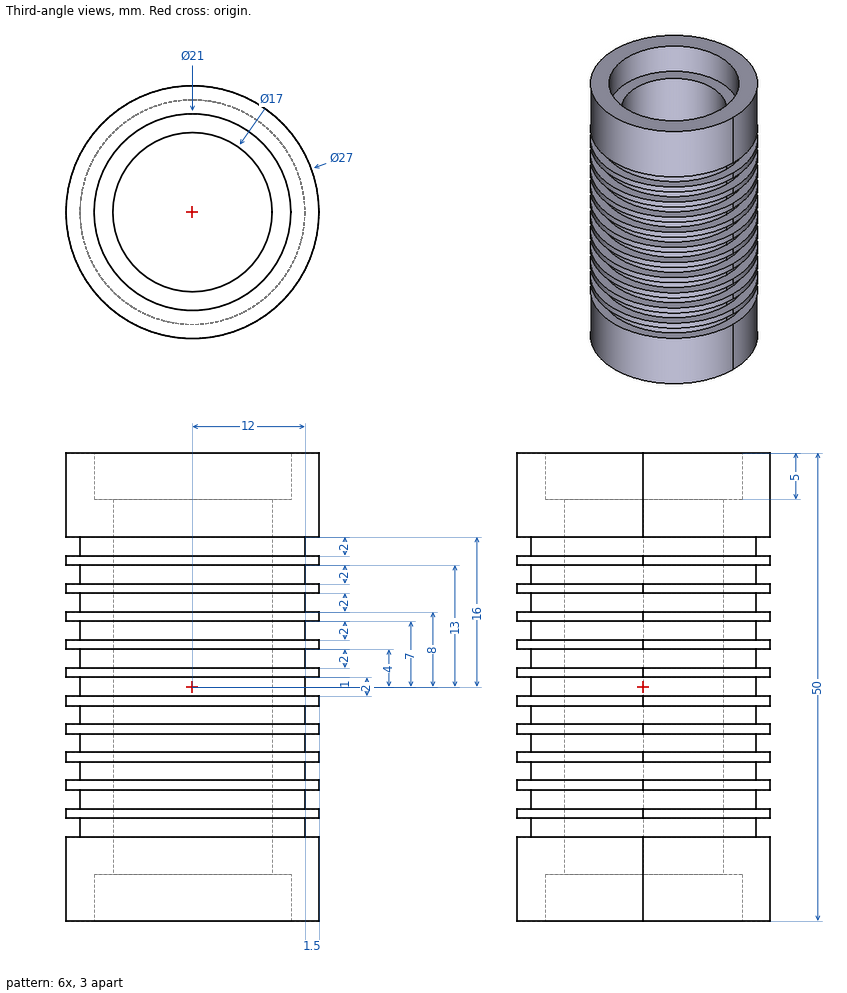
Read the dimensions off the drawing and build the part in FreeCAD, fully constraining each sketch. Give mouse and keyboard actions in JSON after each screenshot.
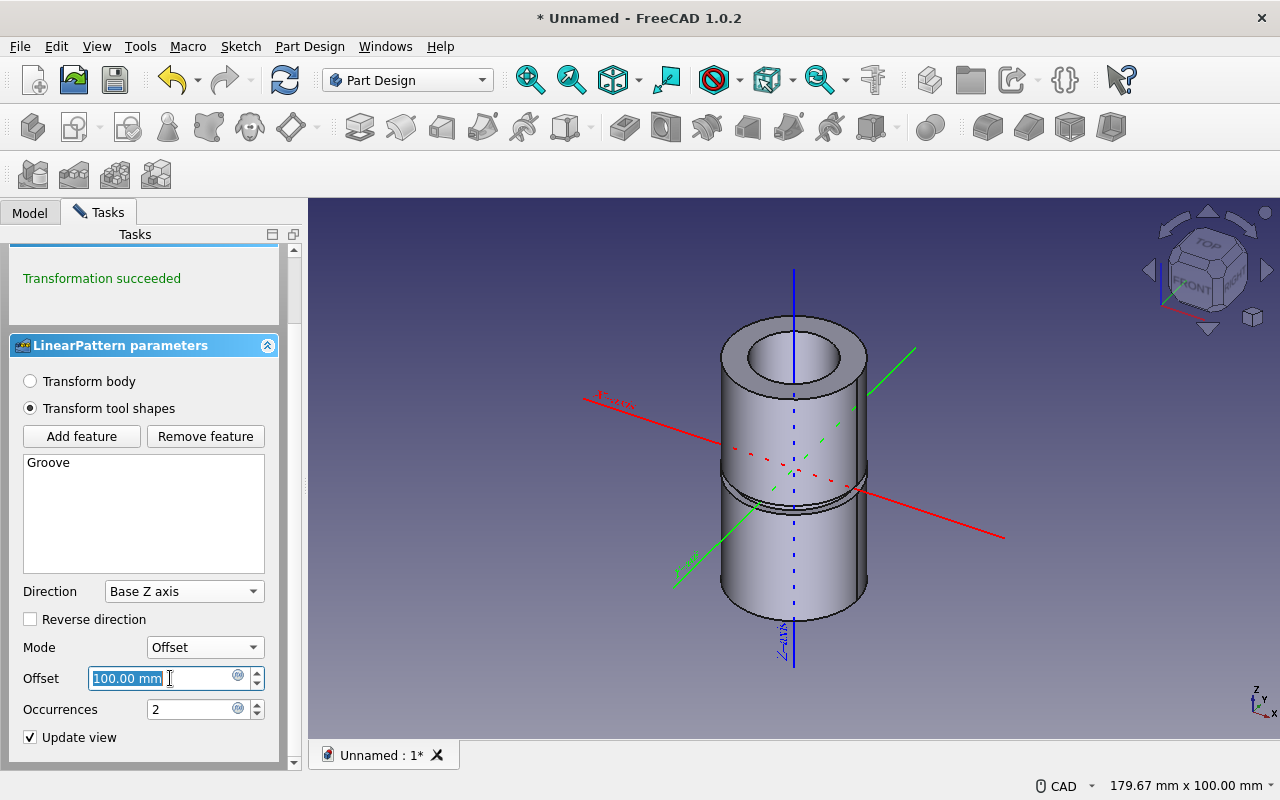
{"action": "type", "text": "3"}
{"action": "key", "text": "Tab"}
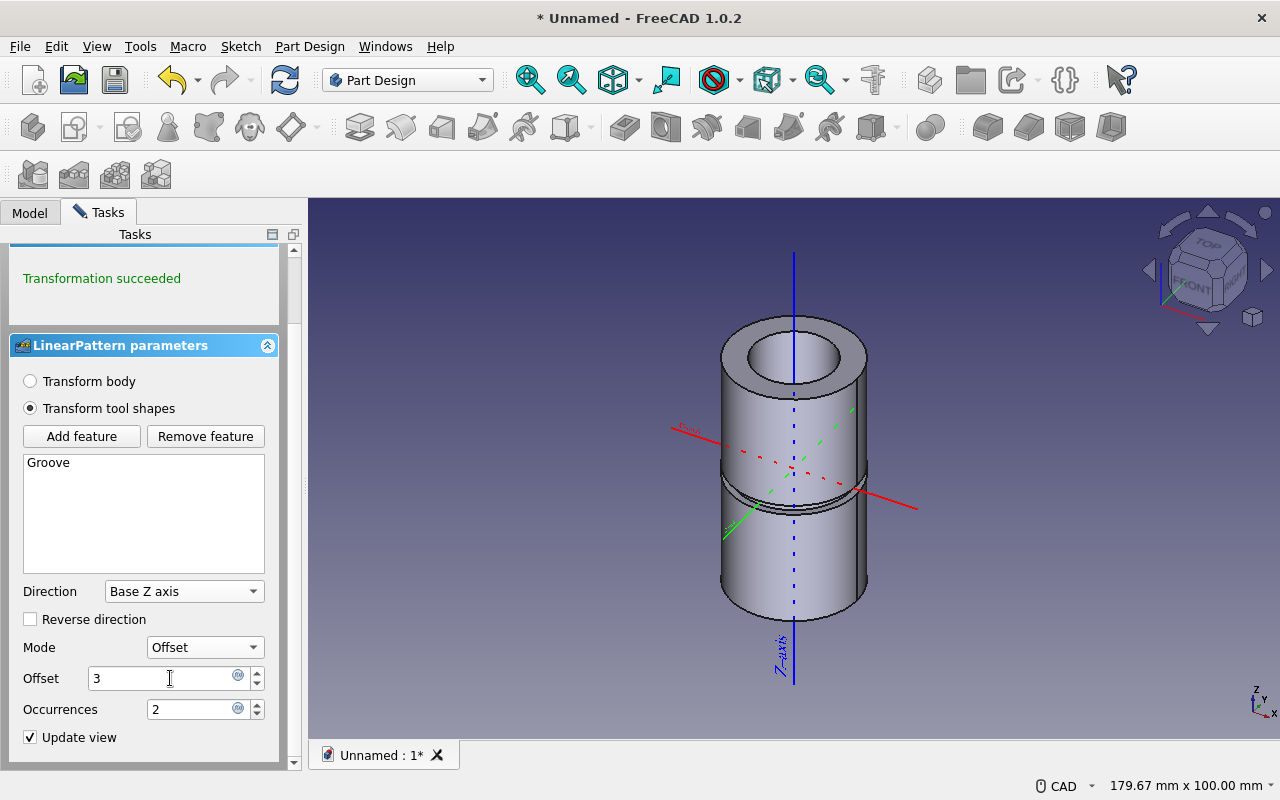
{"action": "triple_click", "coordinate": [199, 710]}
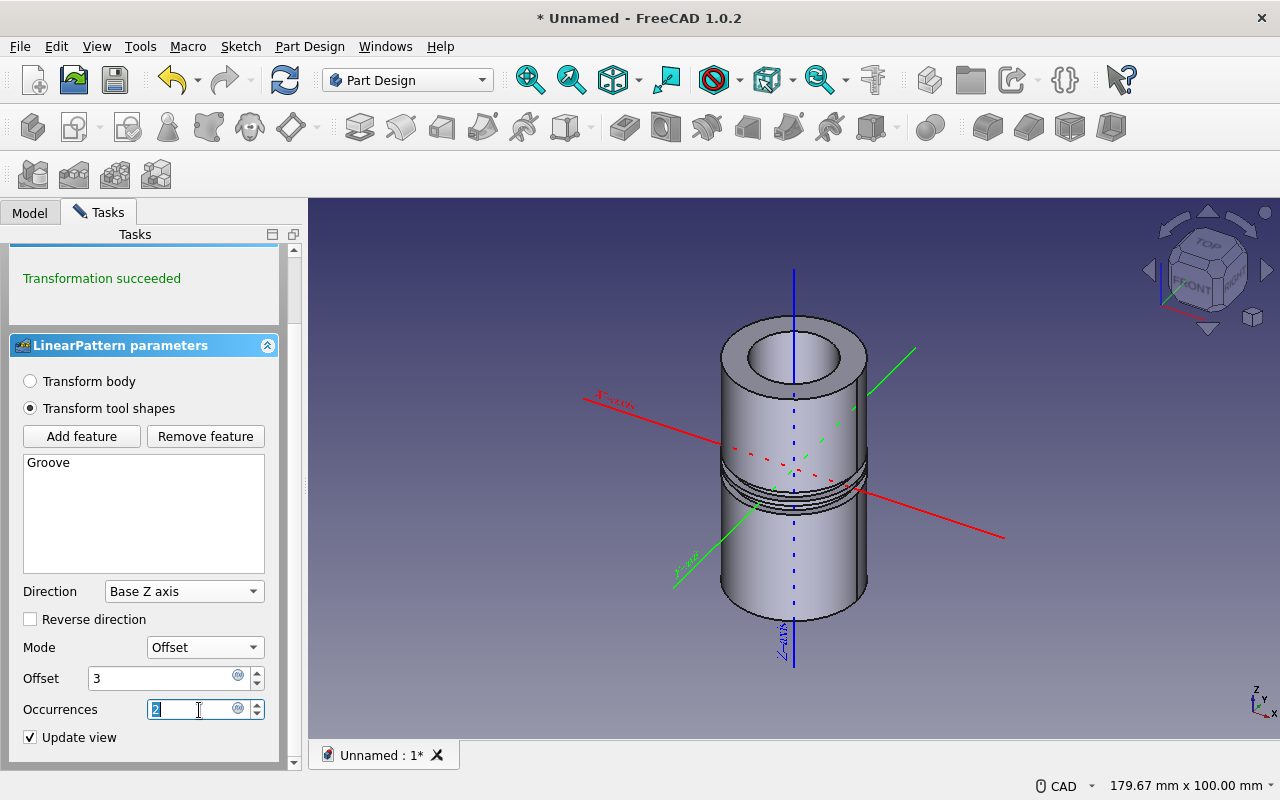
{"action": "type", "text": "6"}
{"action": "key", "text": "Tab"}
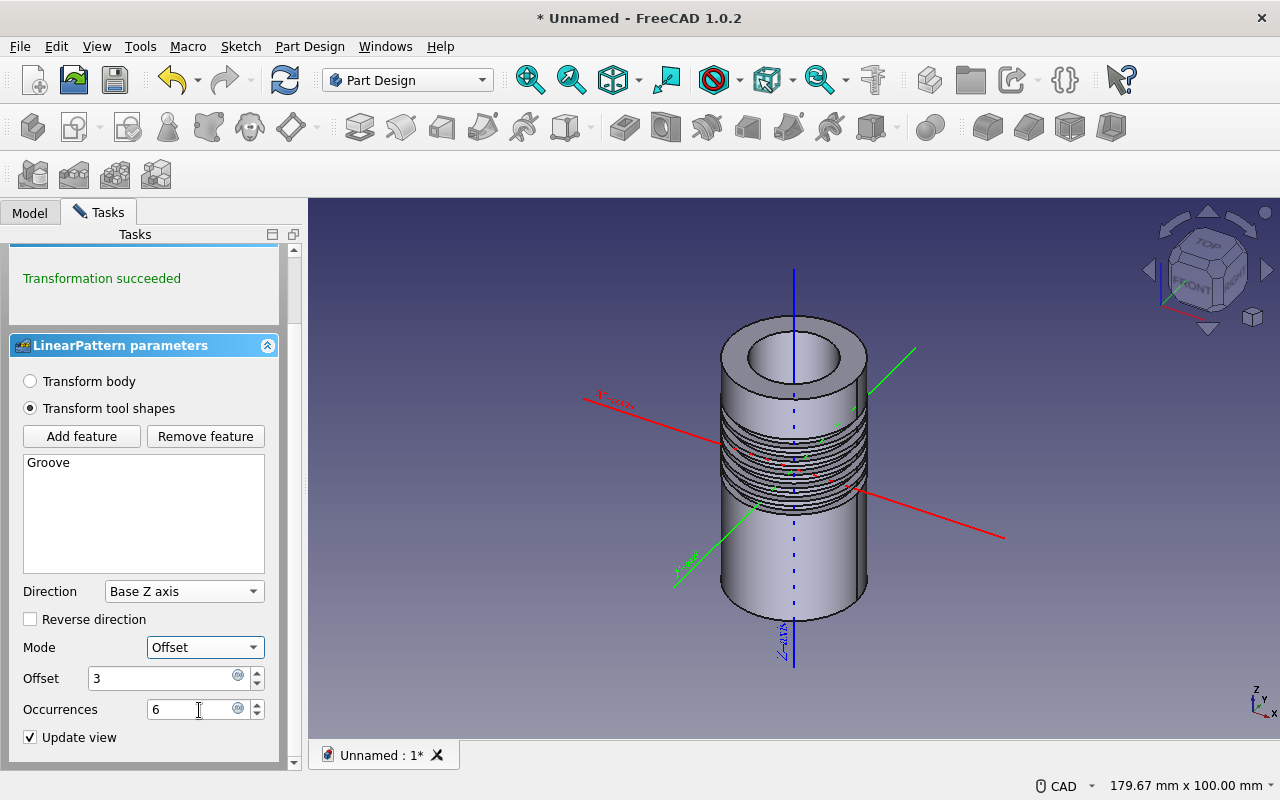
{"action": "left_click", "coordinate": [31, 619]}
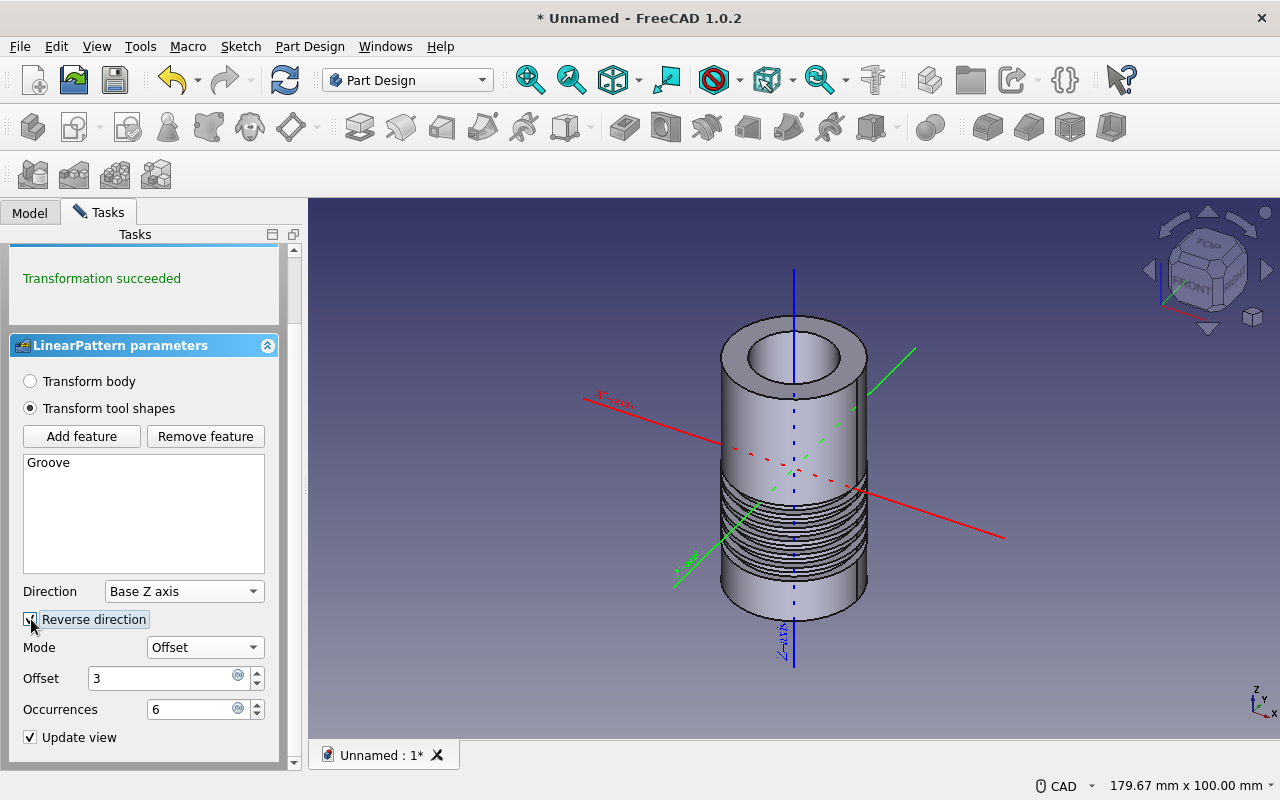
{"action": "scroll", "coordinate": [294, 507], "scroll_direction": "up", "scroll_amount": 3}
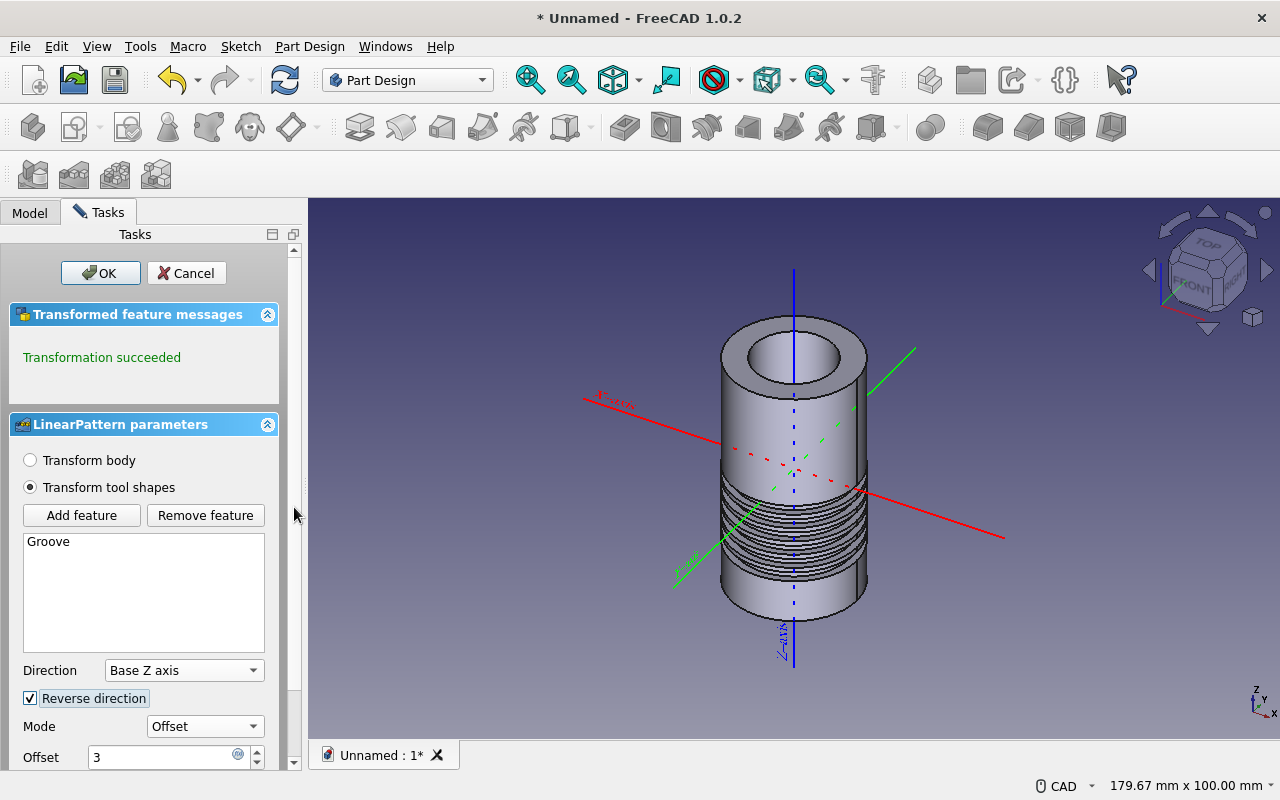
{"action": "left_click", "coordinate": [101, 273]}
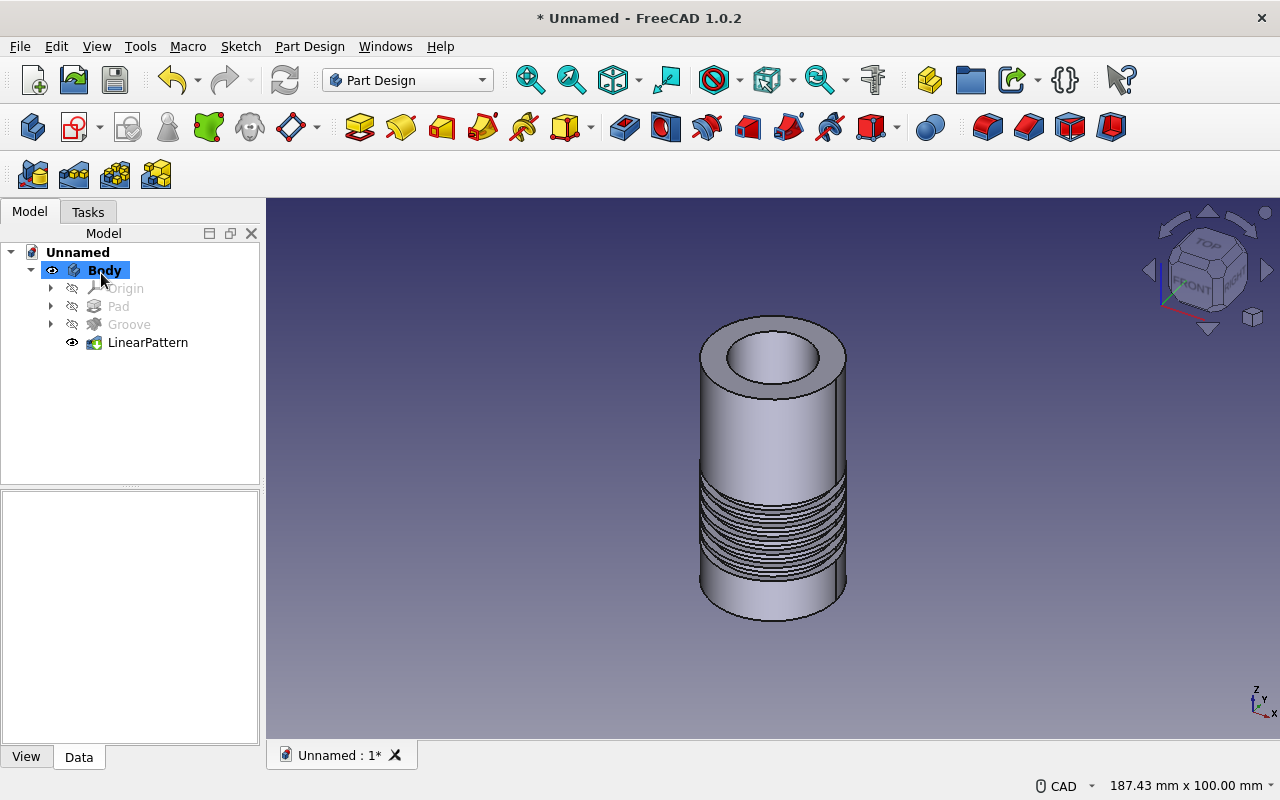
{"action": "left_click", "coordinate": [74, 128]}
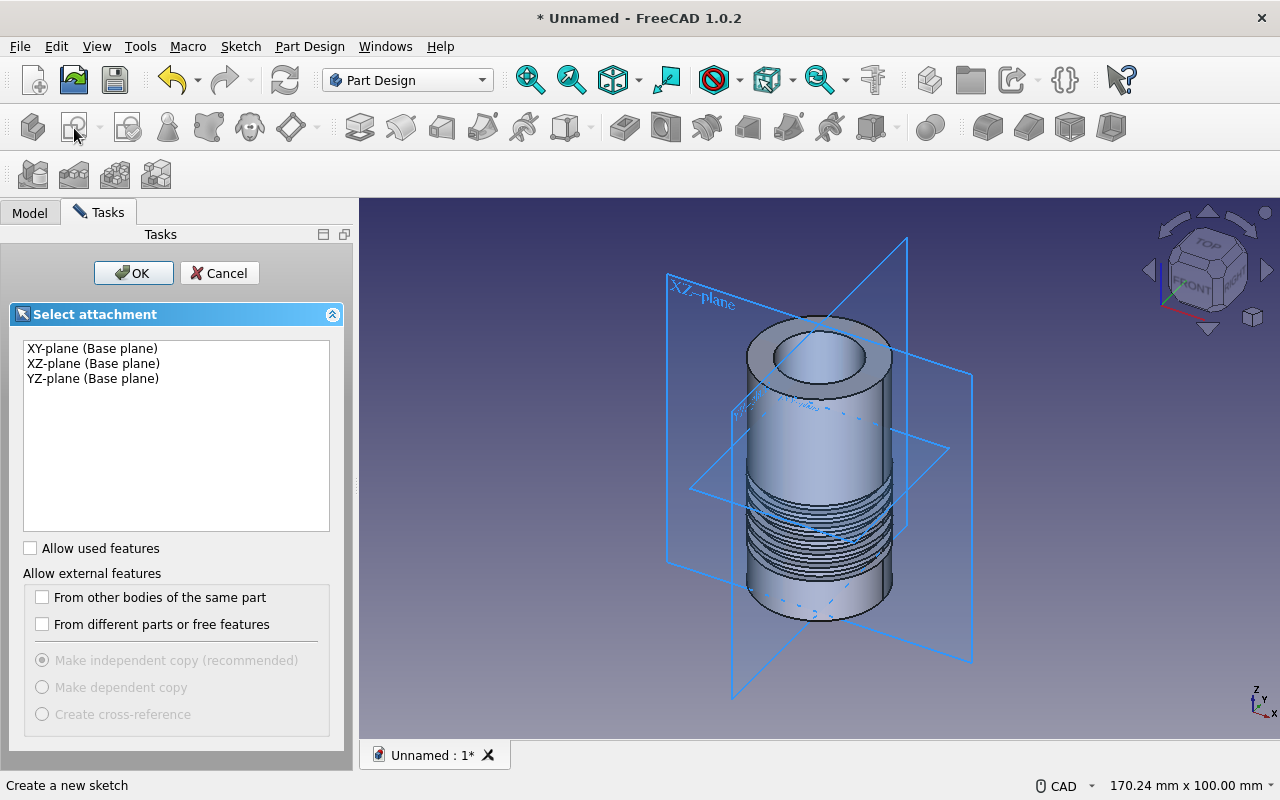
{"action": "left_click", "coordinate": [84, 364]}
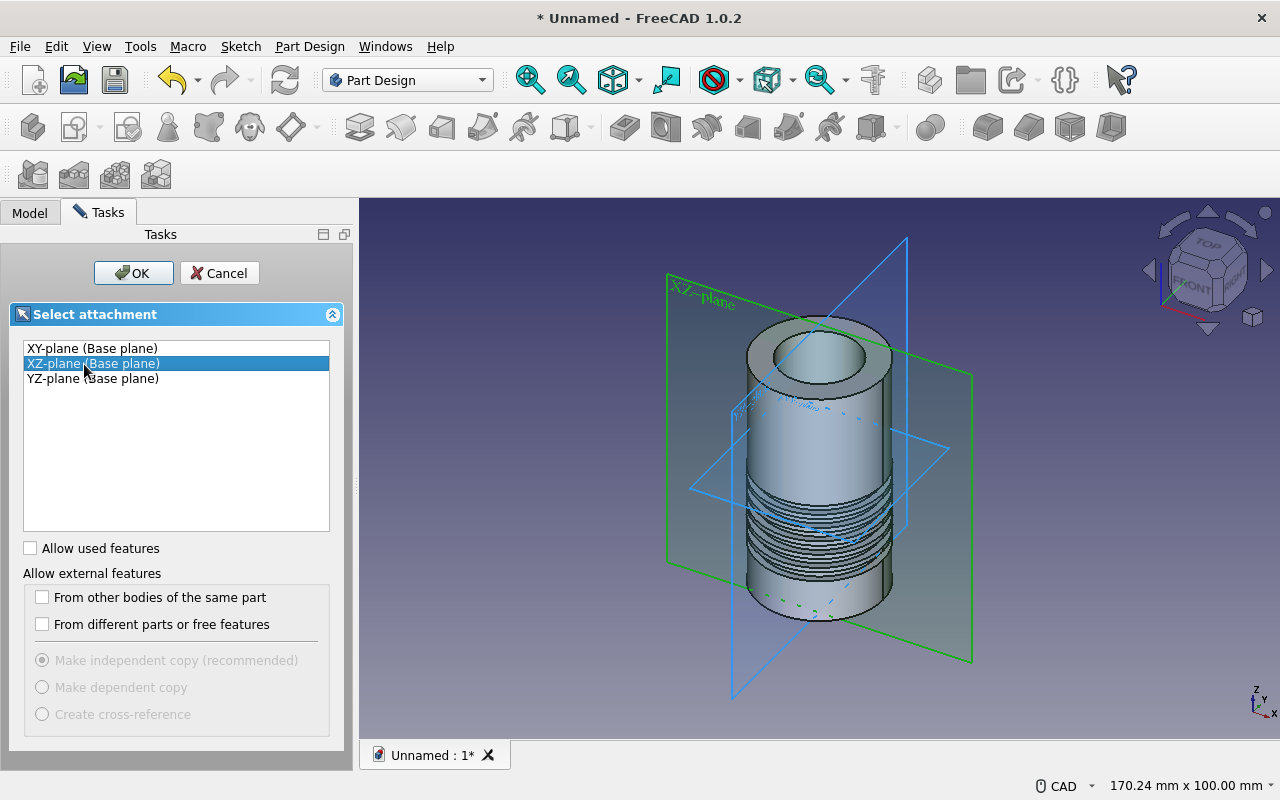
{"action": "left_click", "coordinate": [134, 273]}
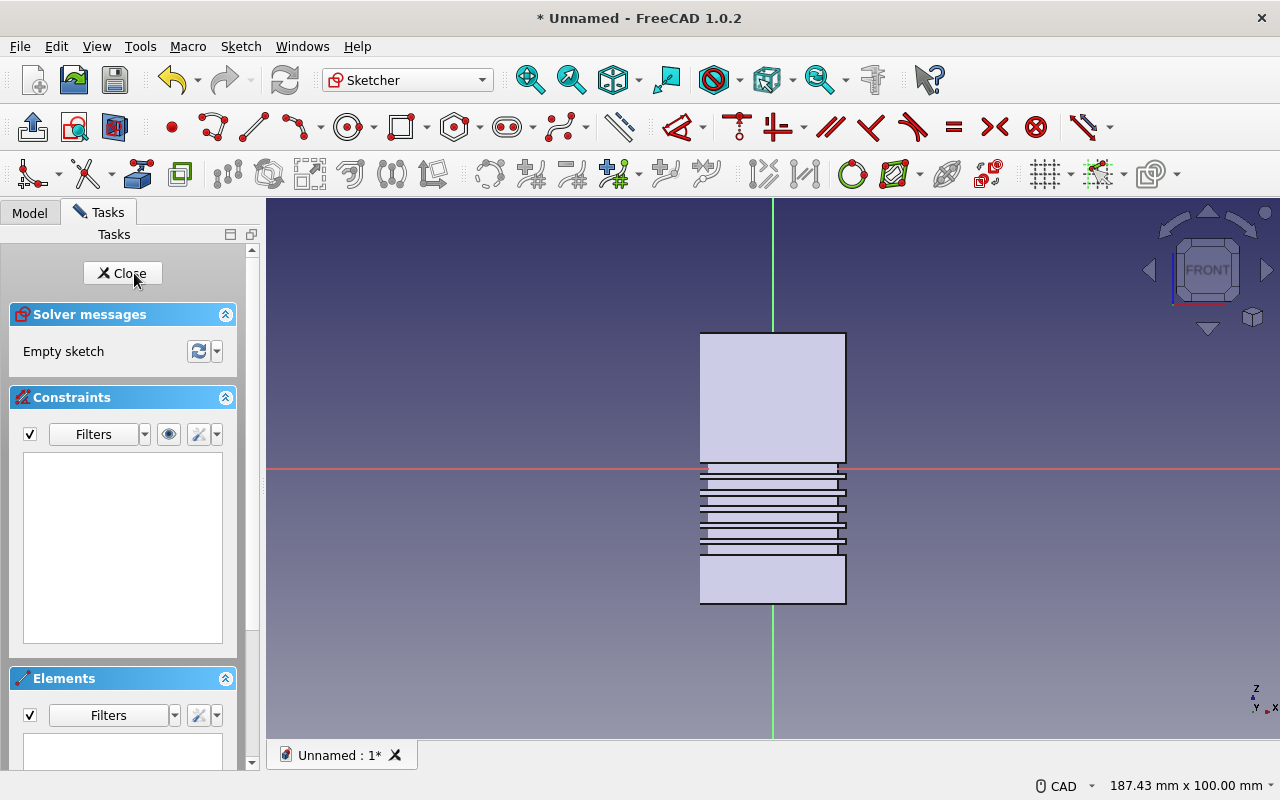
{"action": "left_click", "coordinate": [115, 128]}